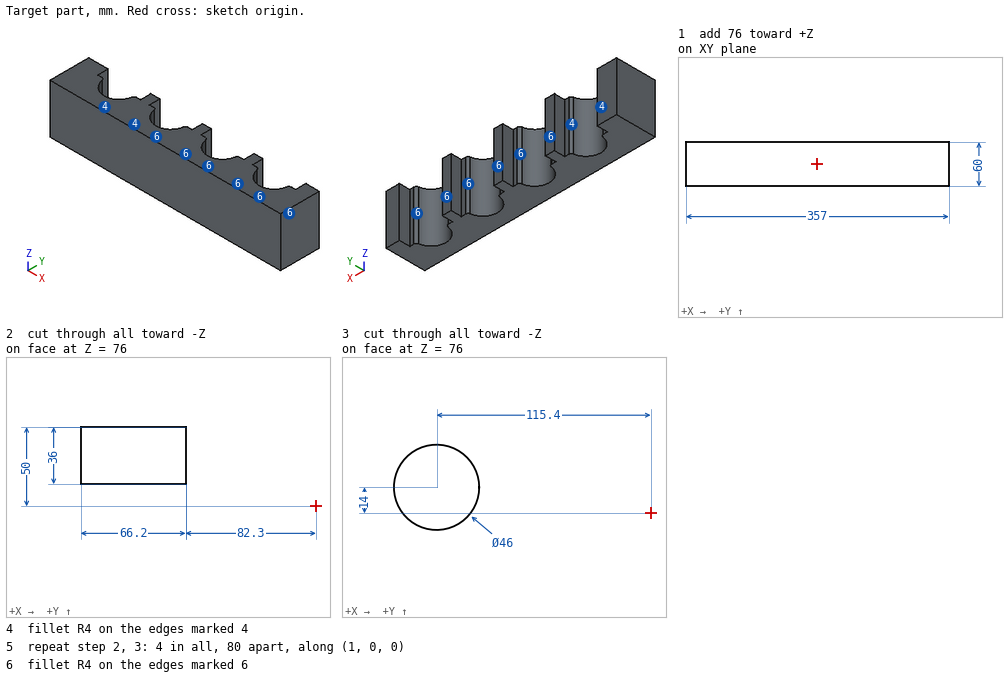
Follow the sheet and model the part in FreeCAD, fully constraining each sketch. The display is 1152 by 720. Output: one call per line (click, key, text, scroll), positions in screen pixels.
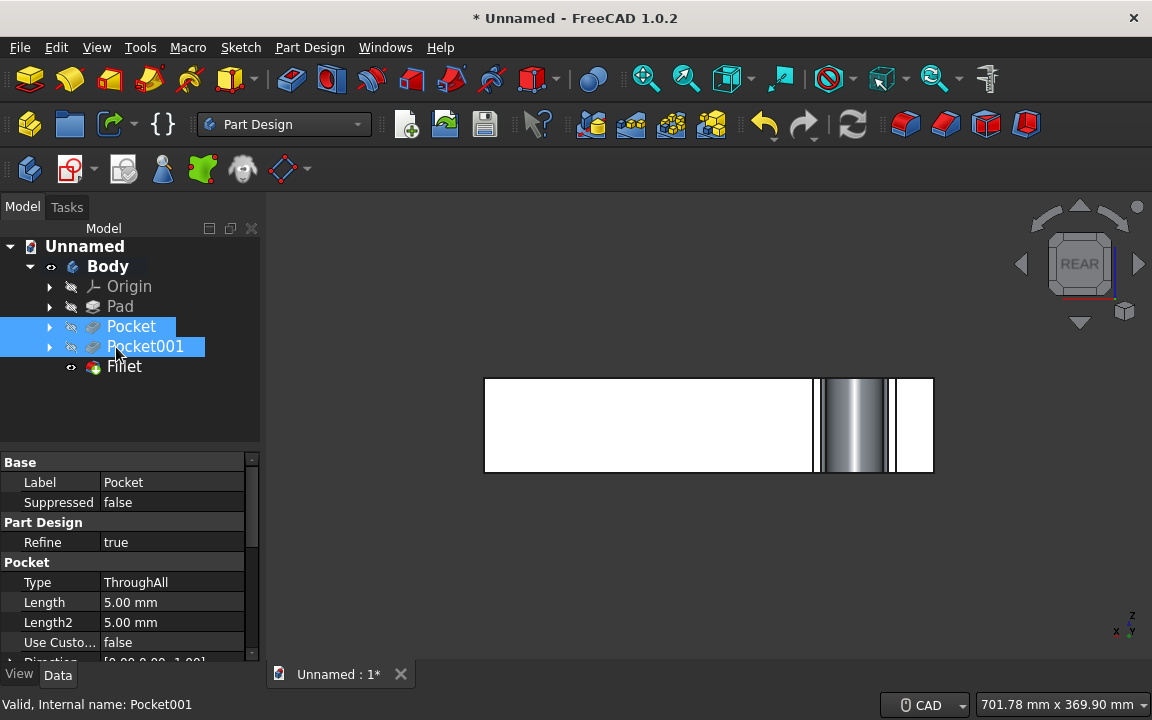
click(632, 124)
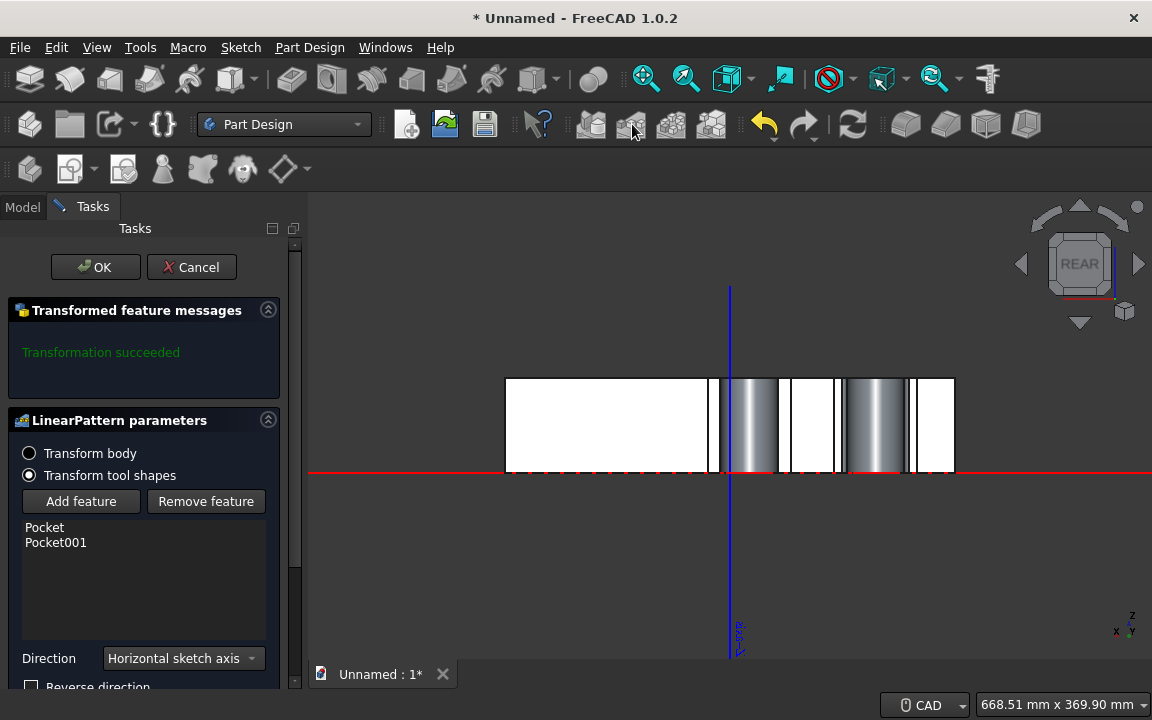
click(184, 658)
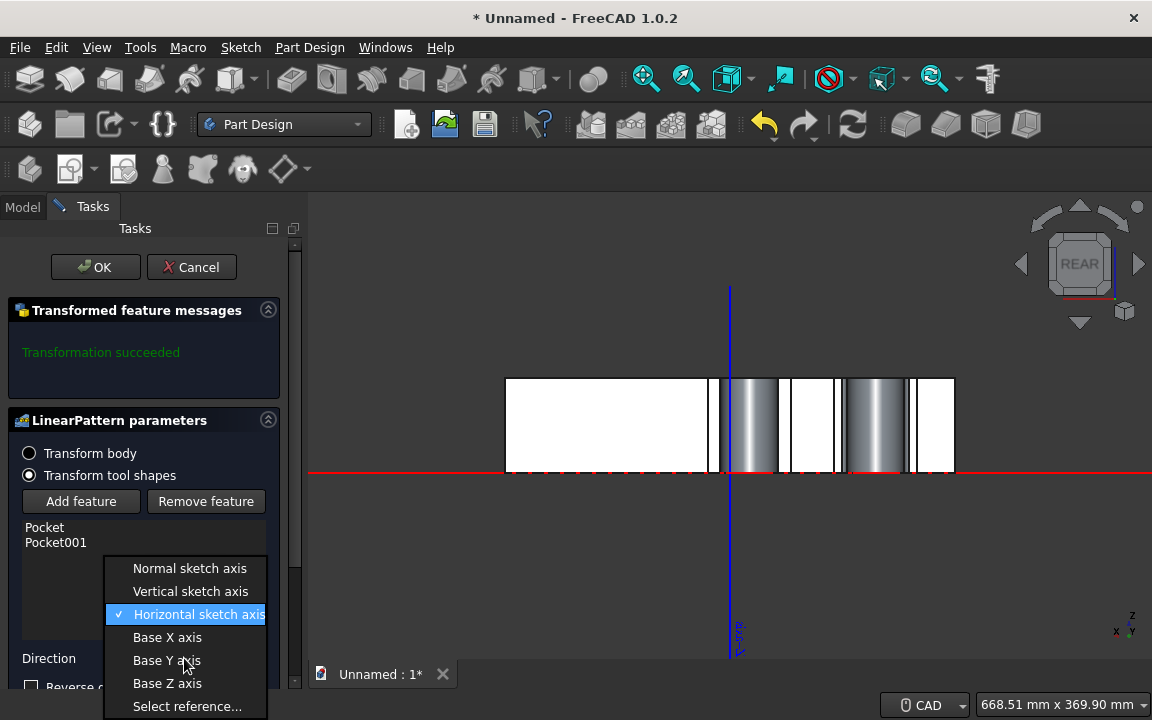
click(184, 638)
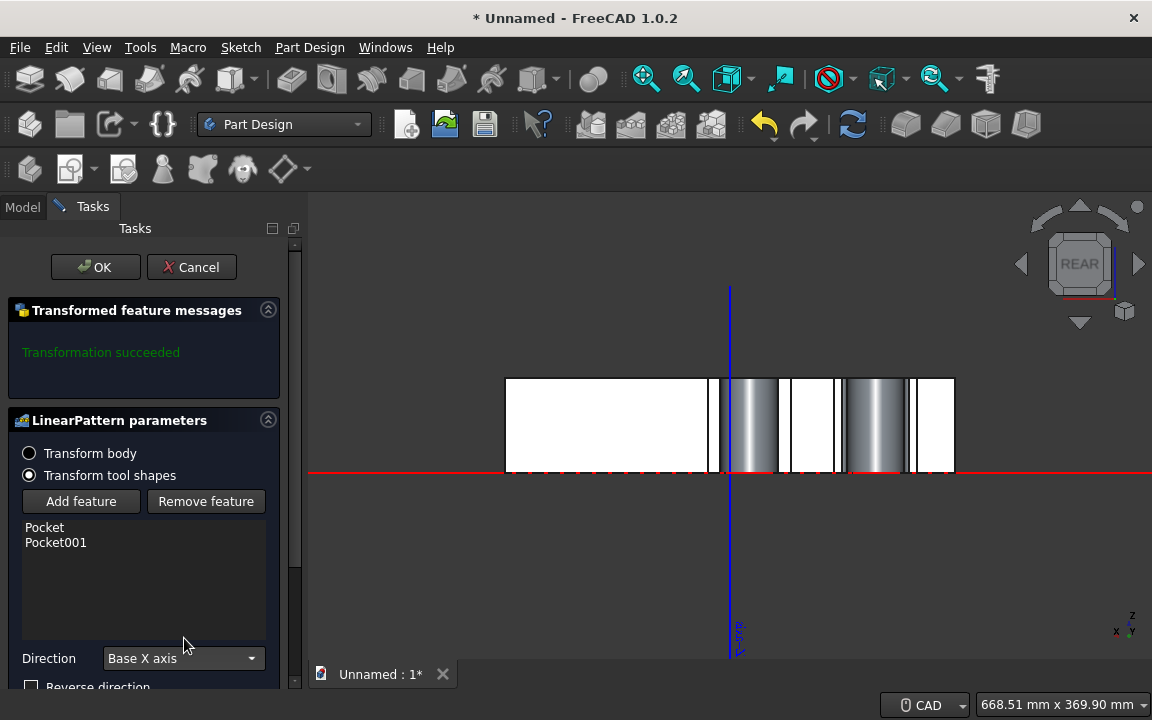
scroll(295, 463, down, 2)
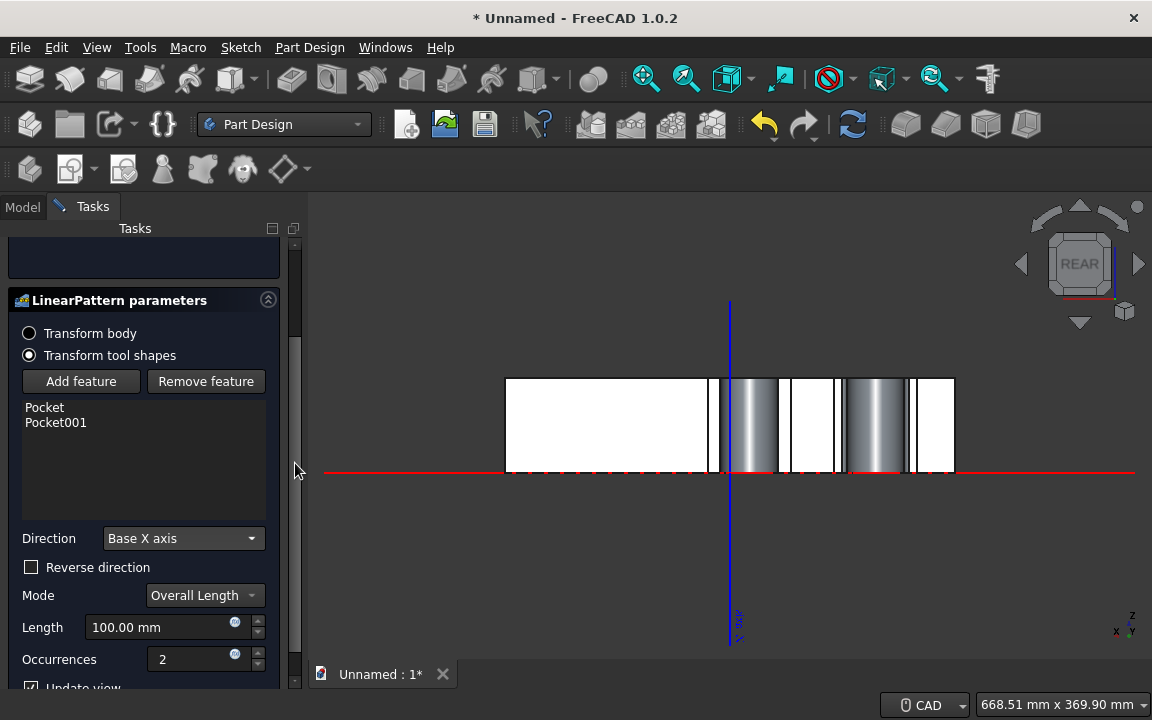
click(206, 596)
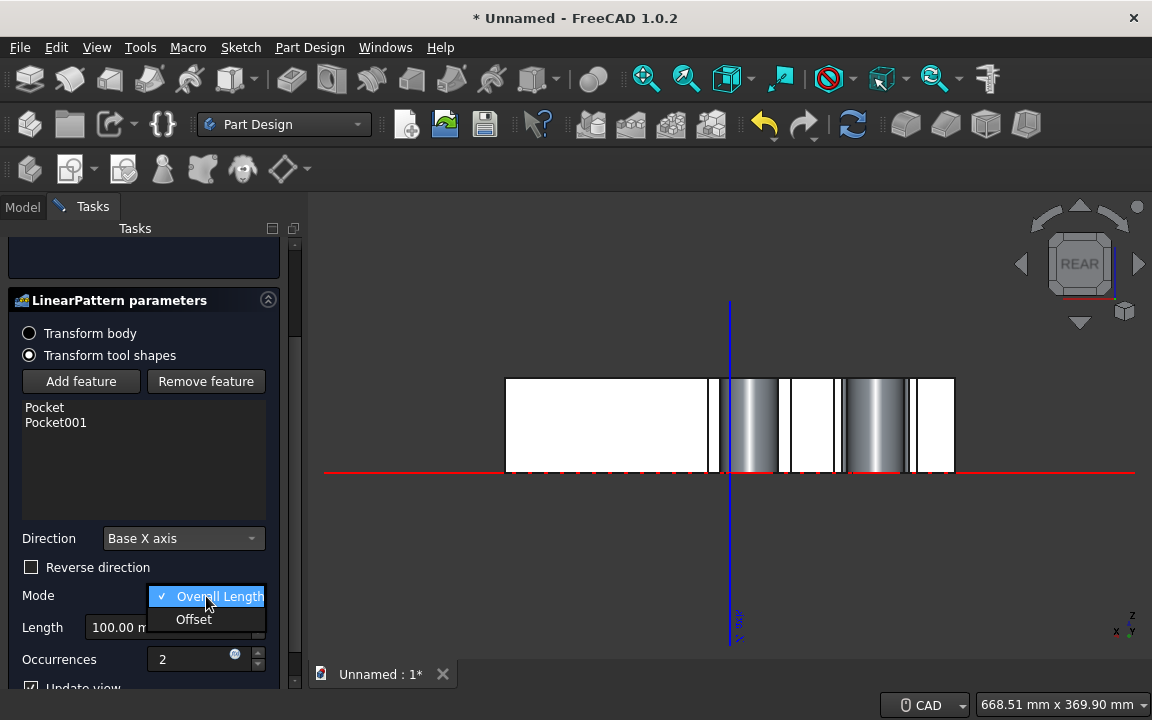
click(206, 620)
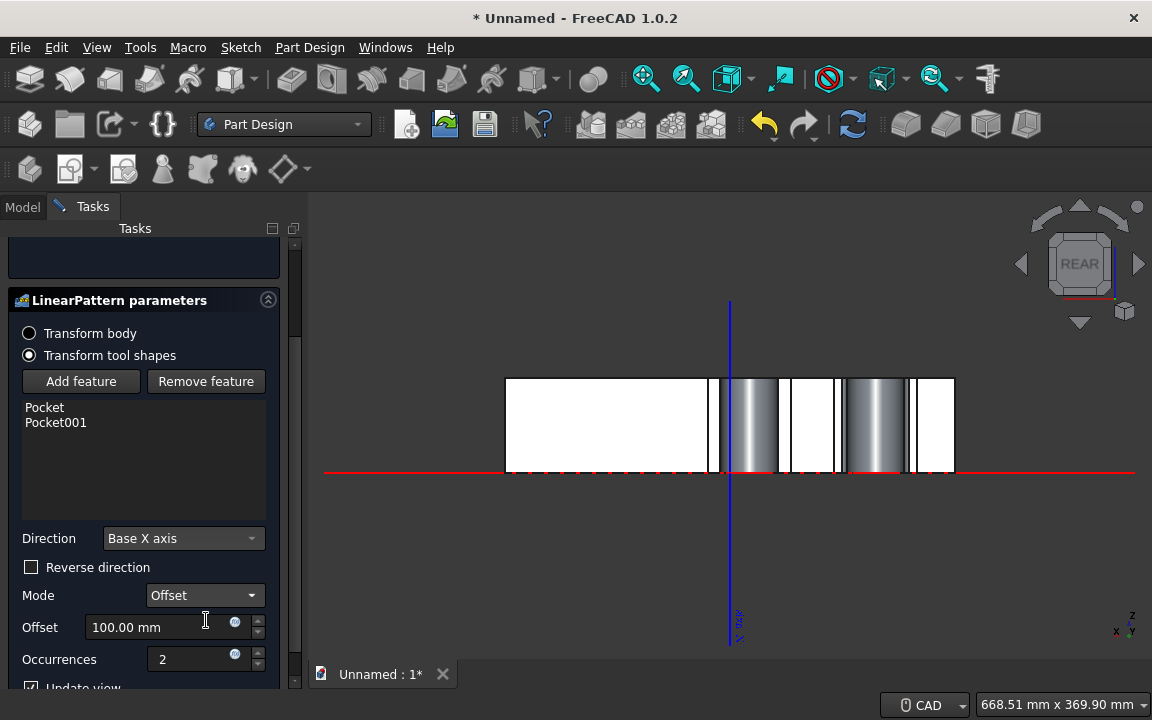
triple_click(168, 627)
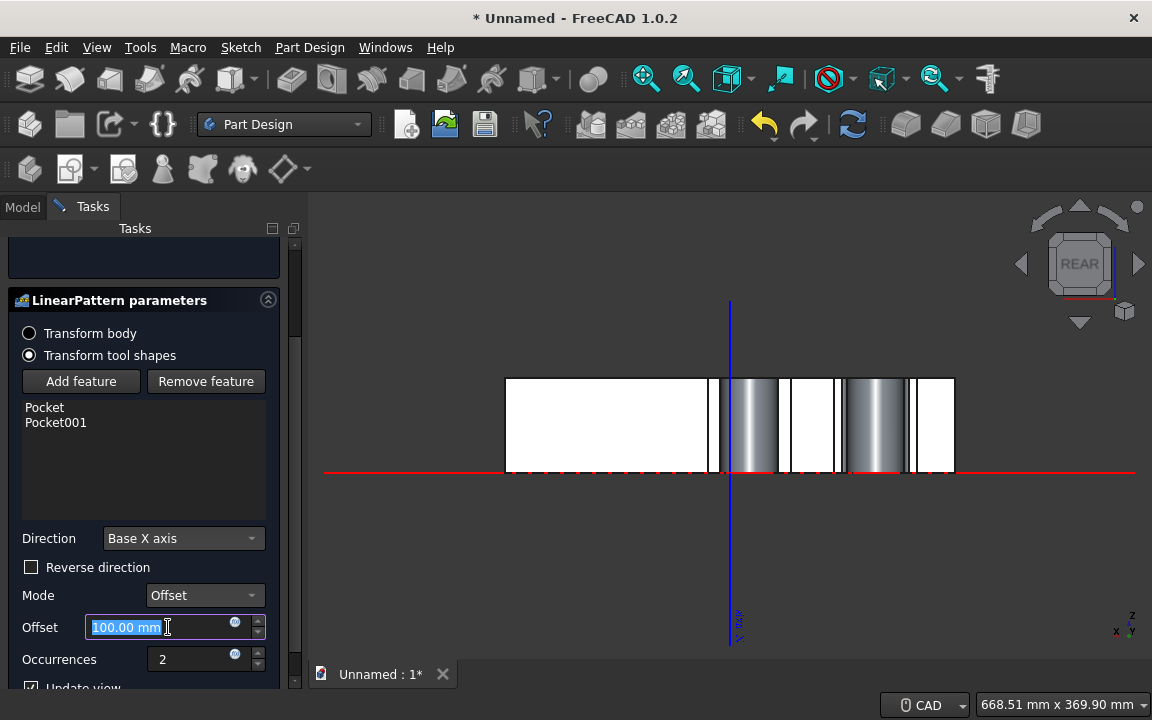
text(80)
key(Tab)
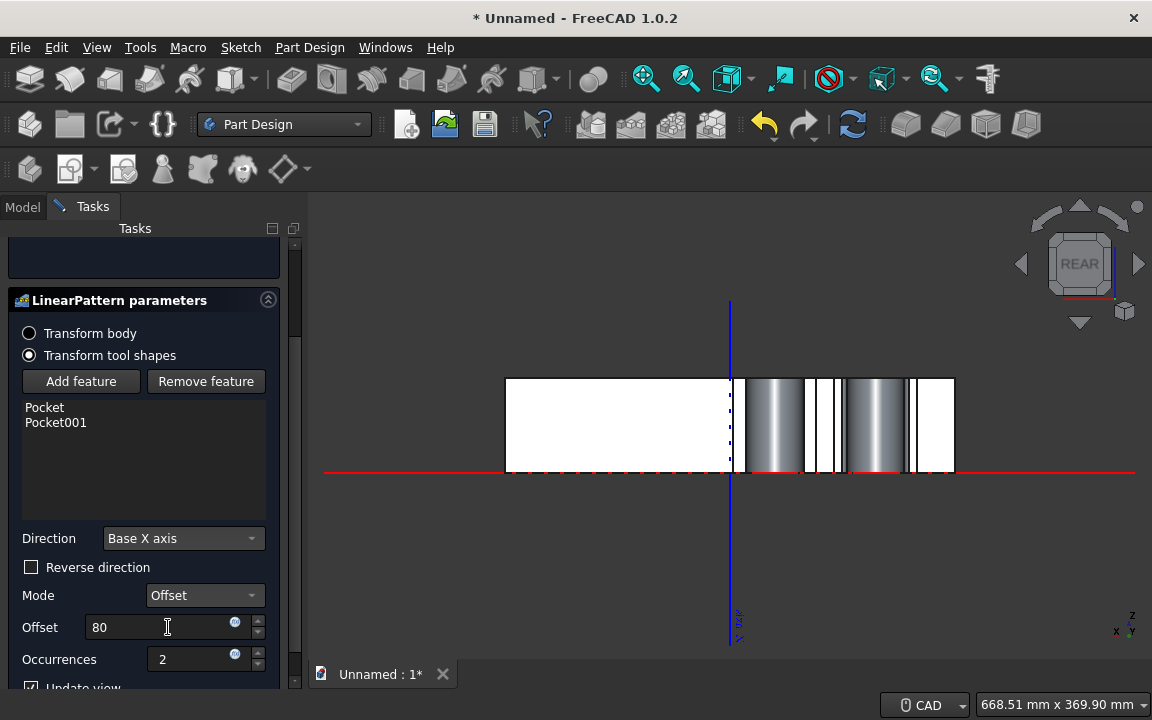
triple_click(198, 659)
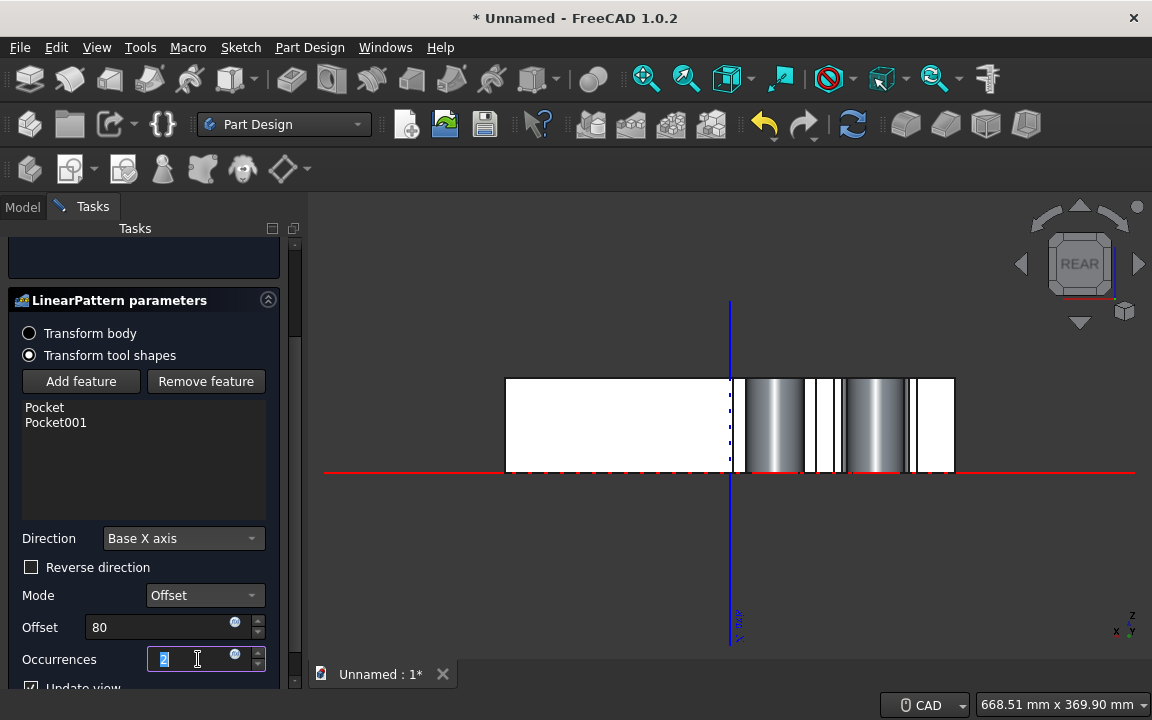
text(4)
key(Tab)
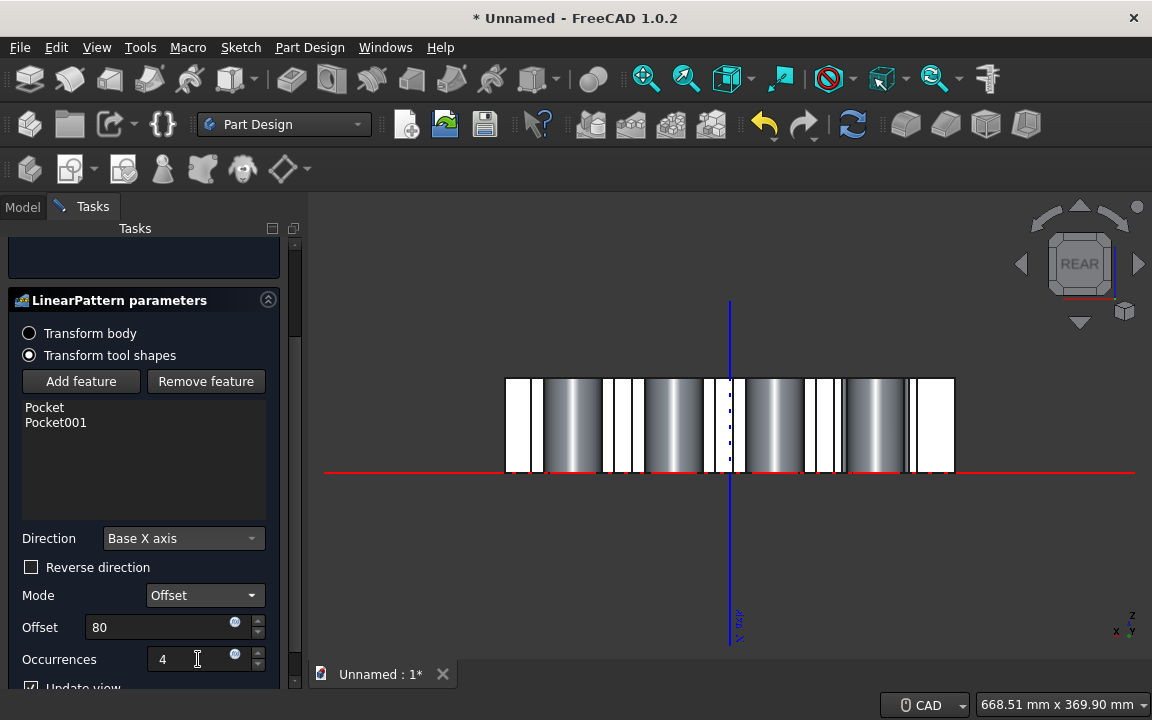
scroll(295, 463, up, 3)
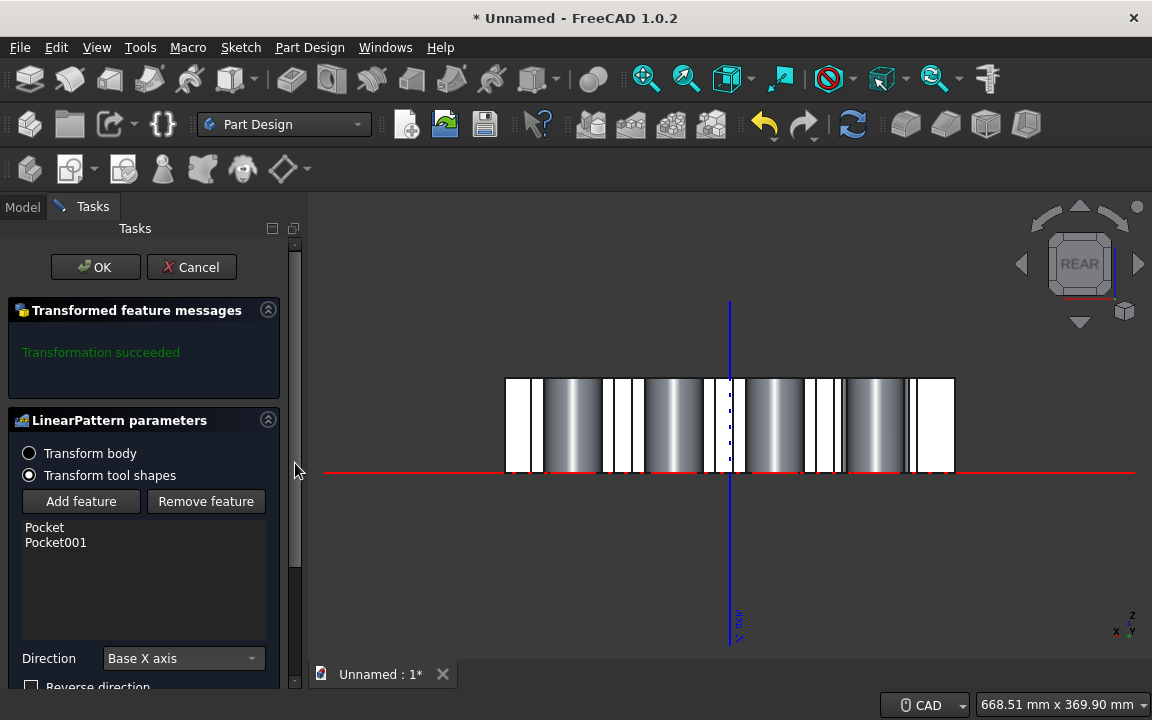
click(96, 267)